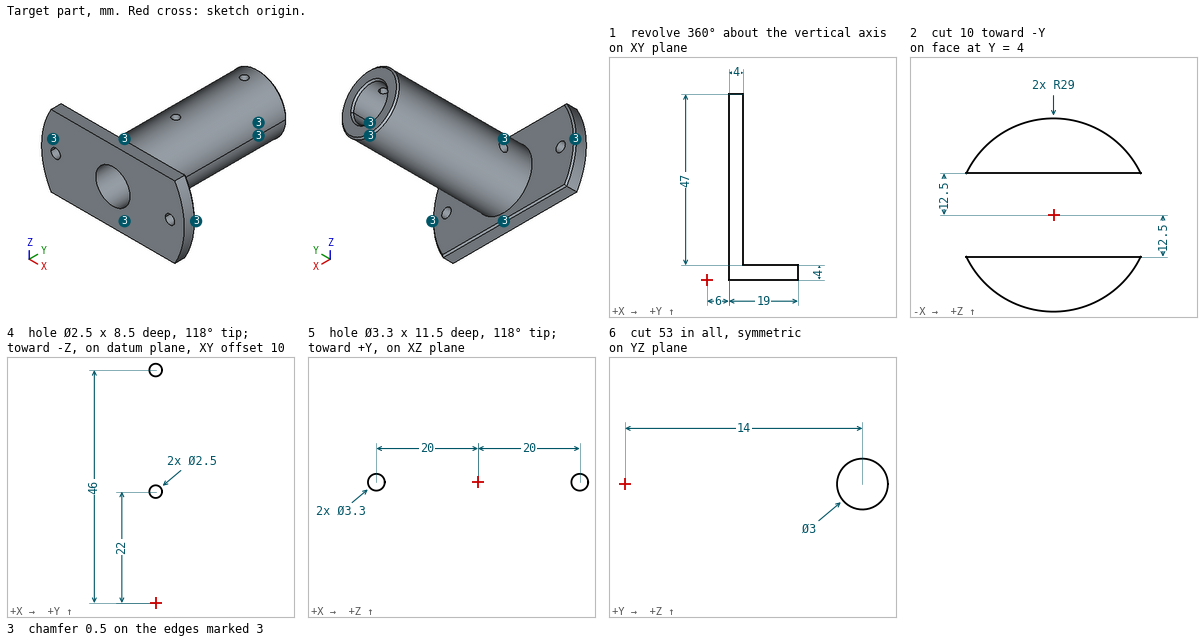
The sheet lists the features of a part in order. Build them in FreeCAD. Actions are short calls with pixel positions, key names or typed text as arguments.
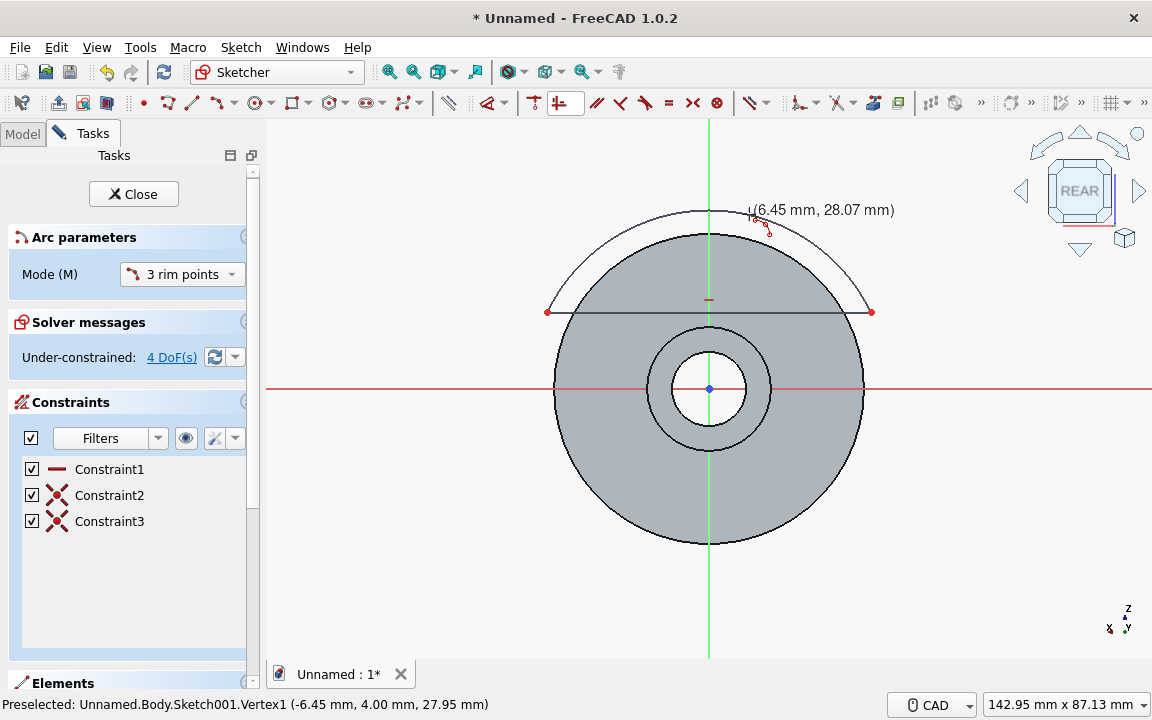
click(192, 104)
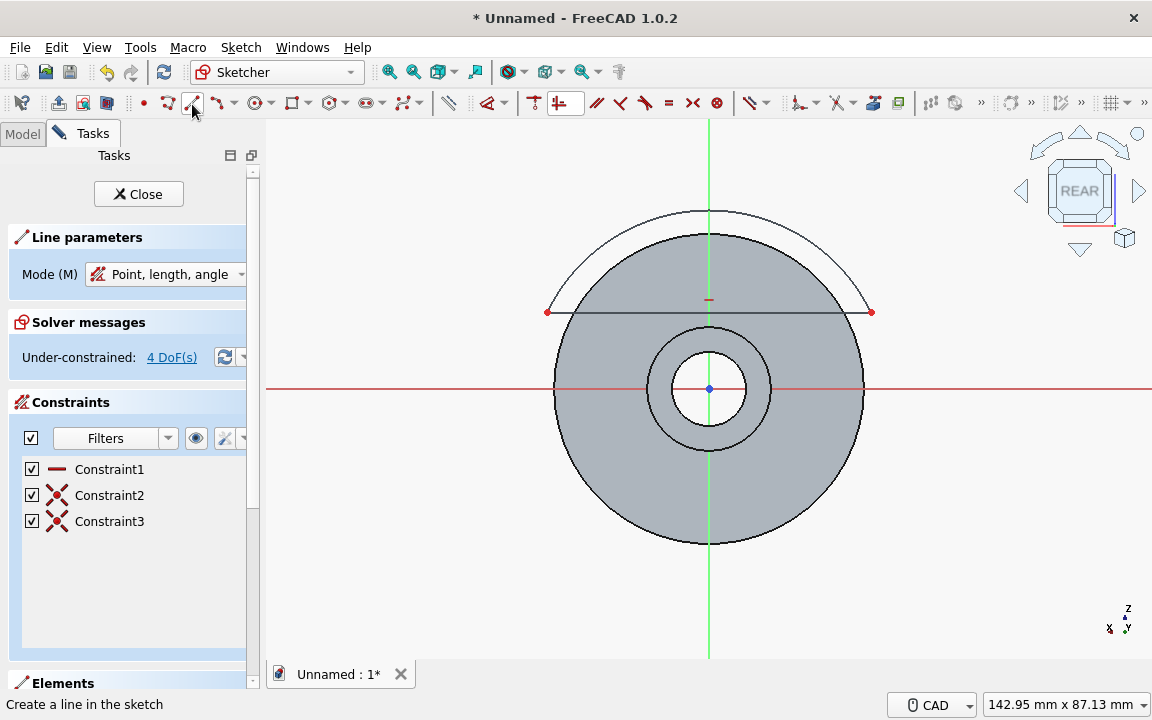
click(871, 466)
click(547, 466)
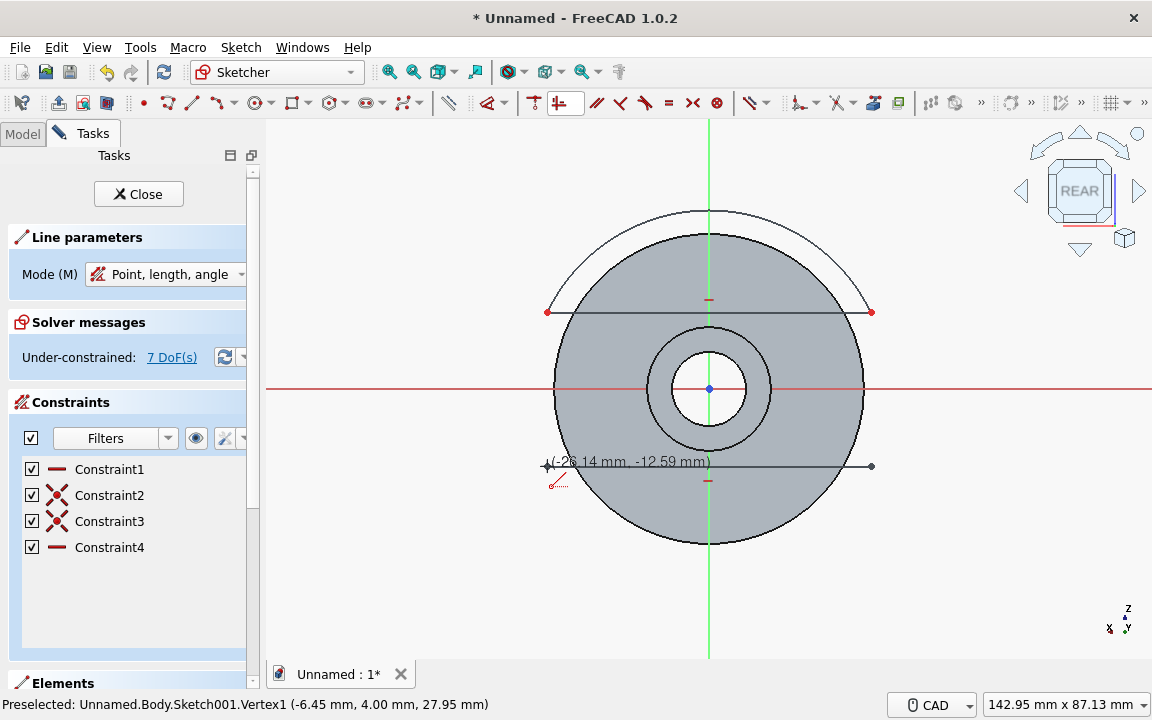
click(218, 104)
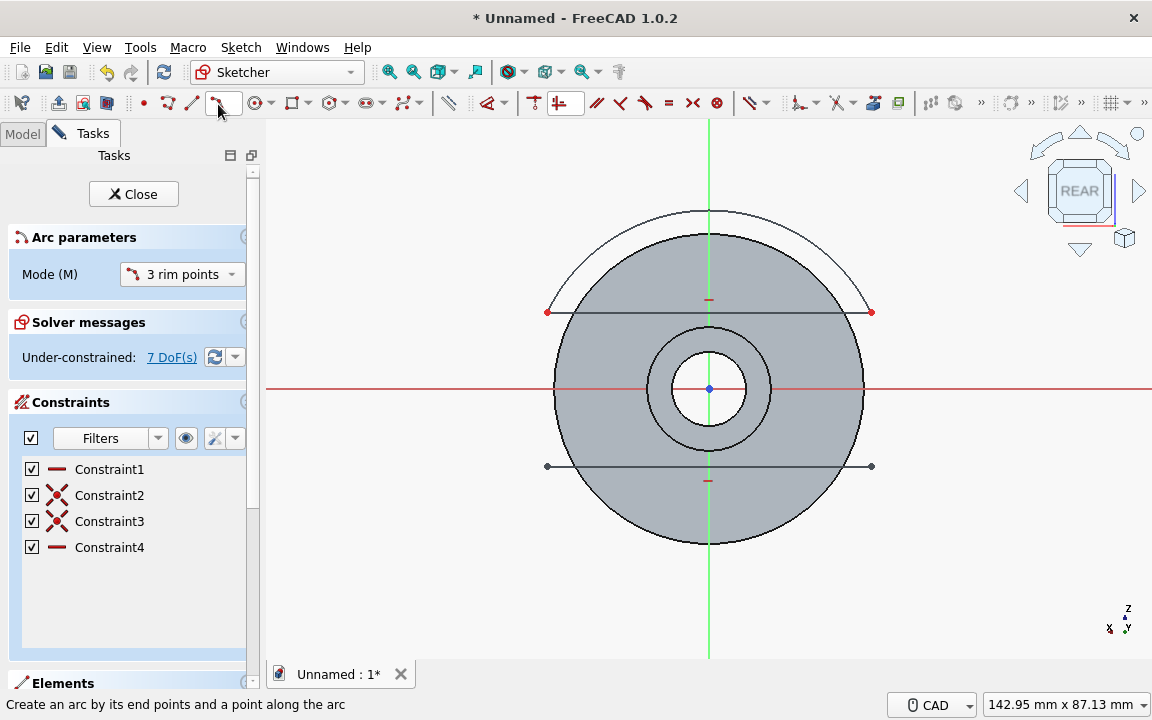
click(547, 467)
click(871, 467)
click(669, 564)
key(Escape)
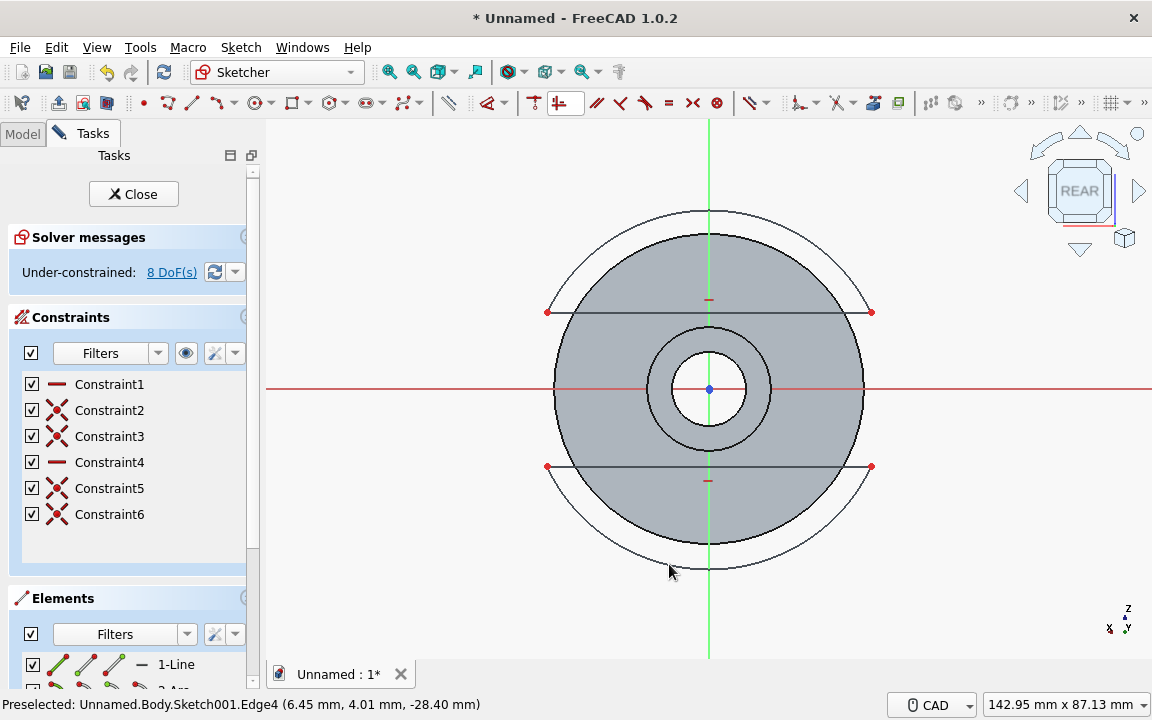
click(787, 228)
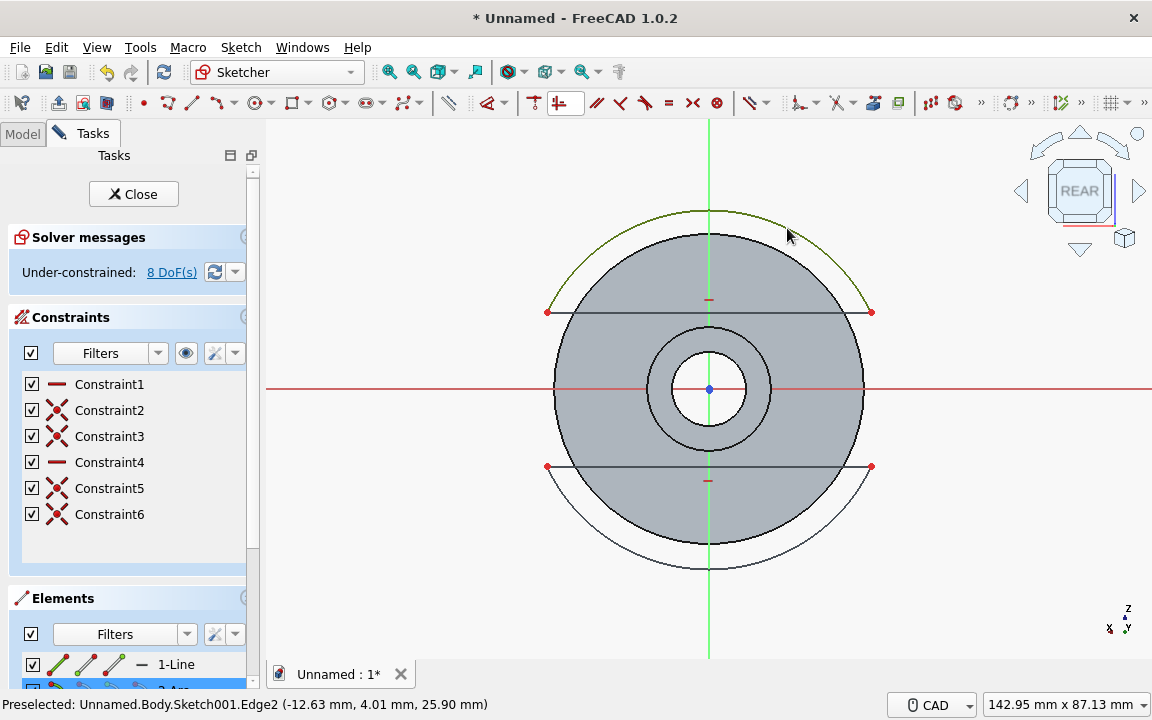
click(631, 552)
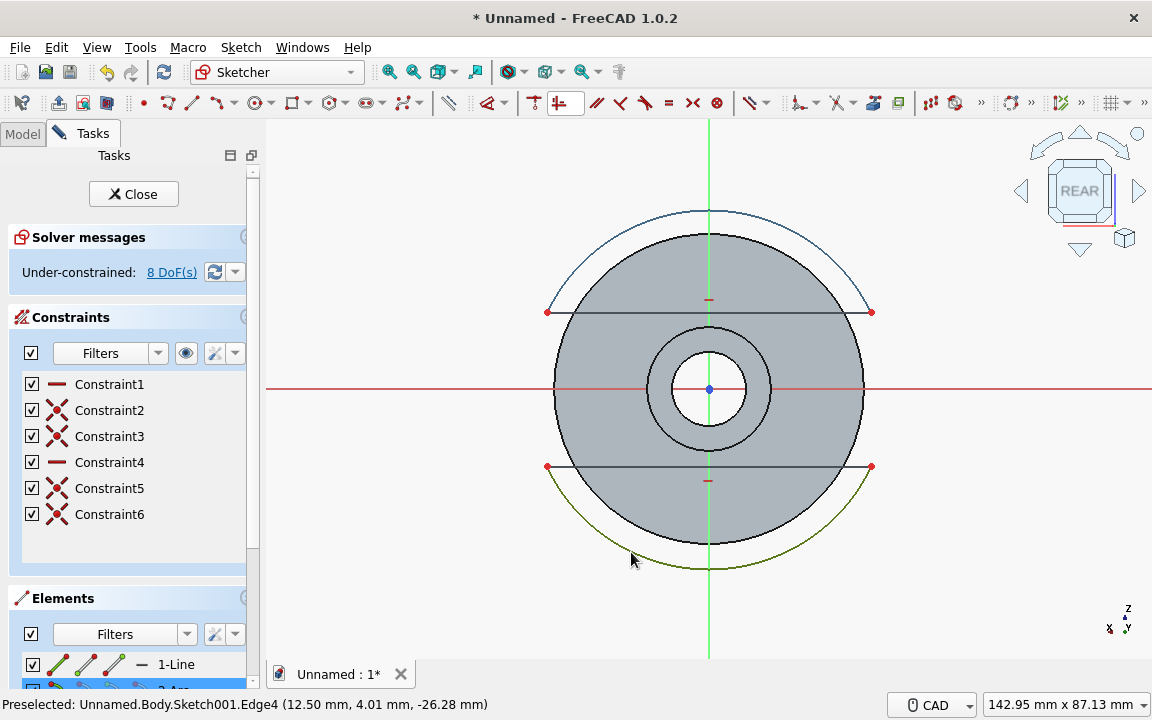
click(534, 104)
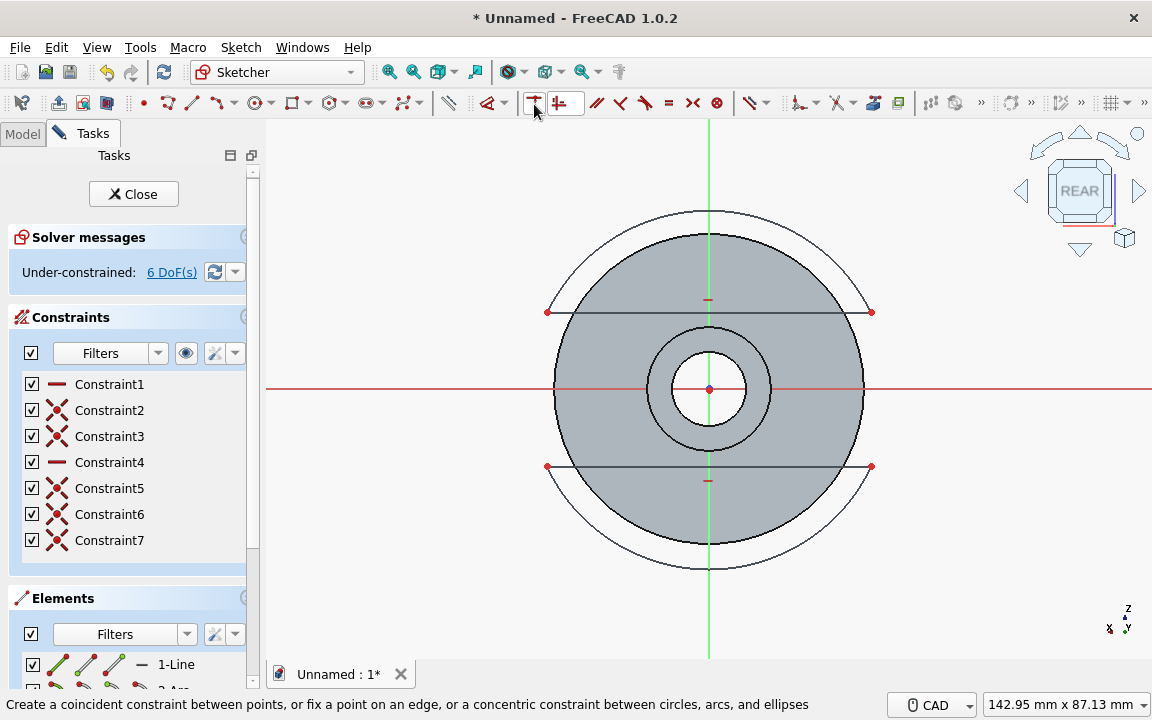
drag(699, 379, 719, 400)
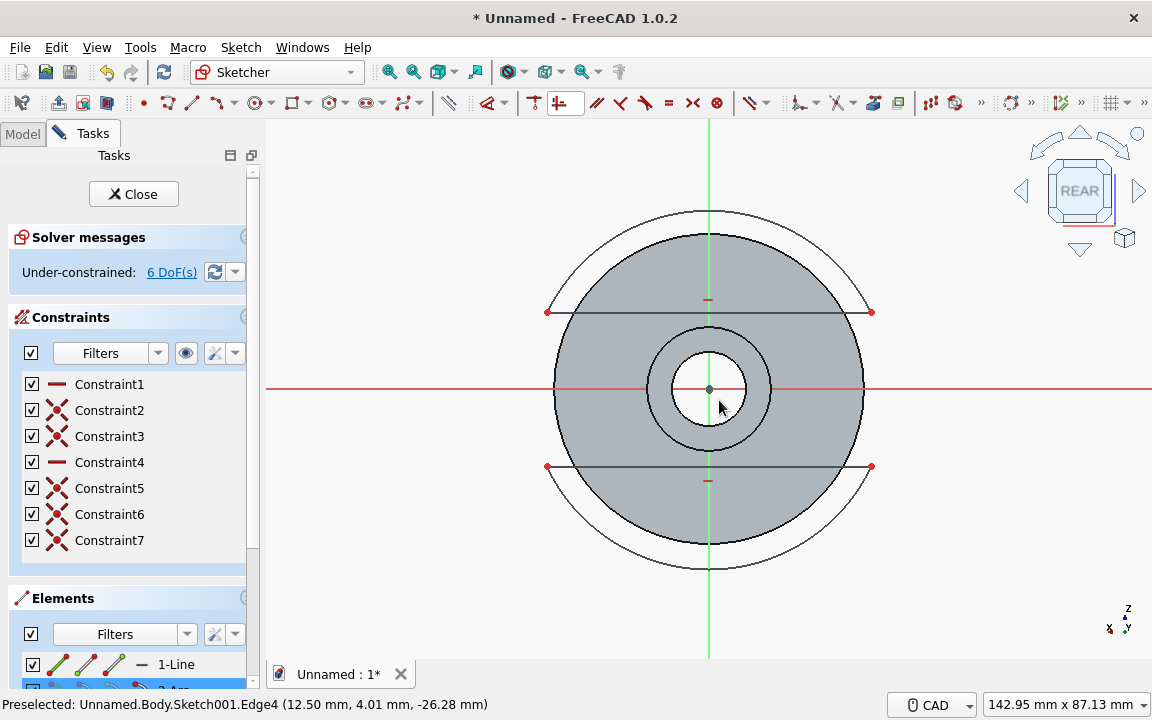
click(534, 104)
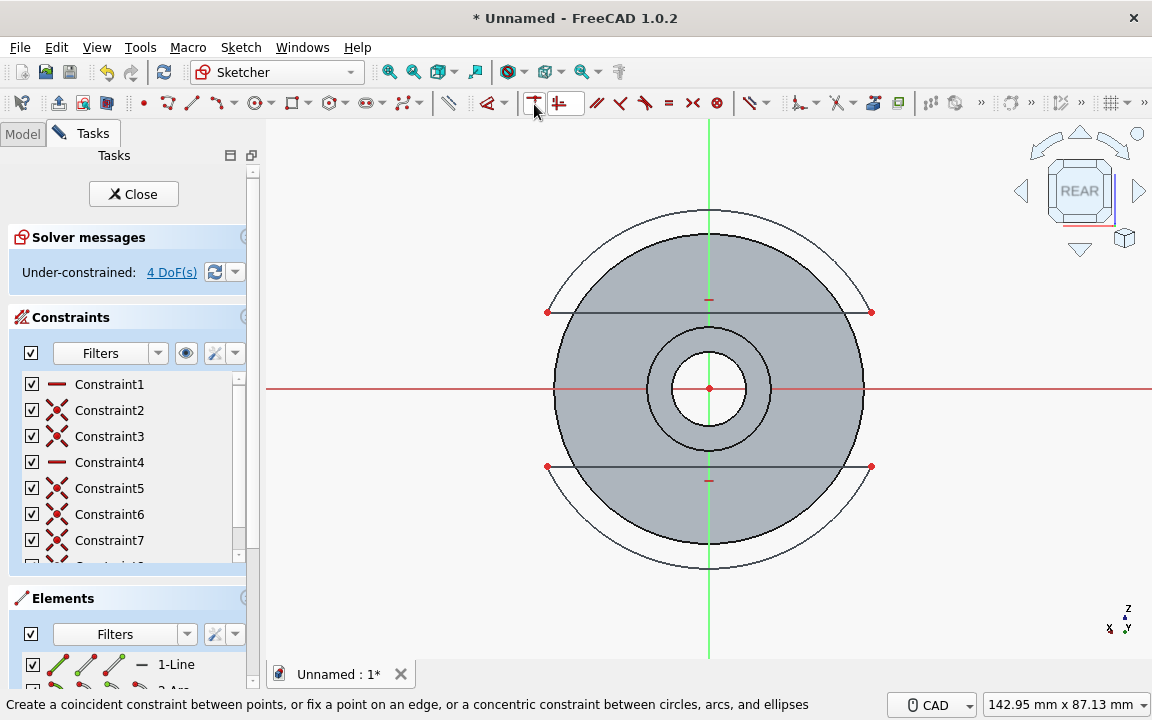
click(787, 228)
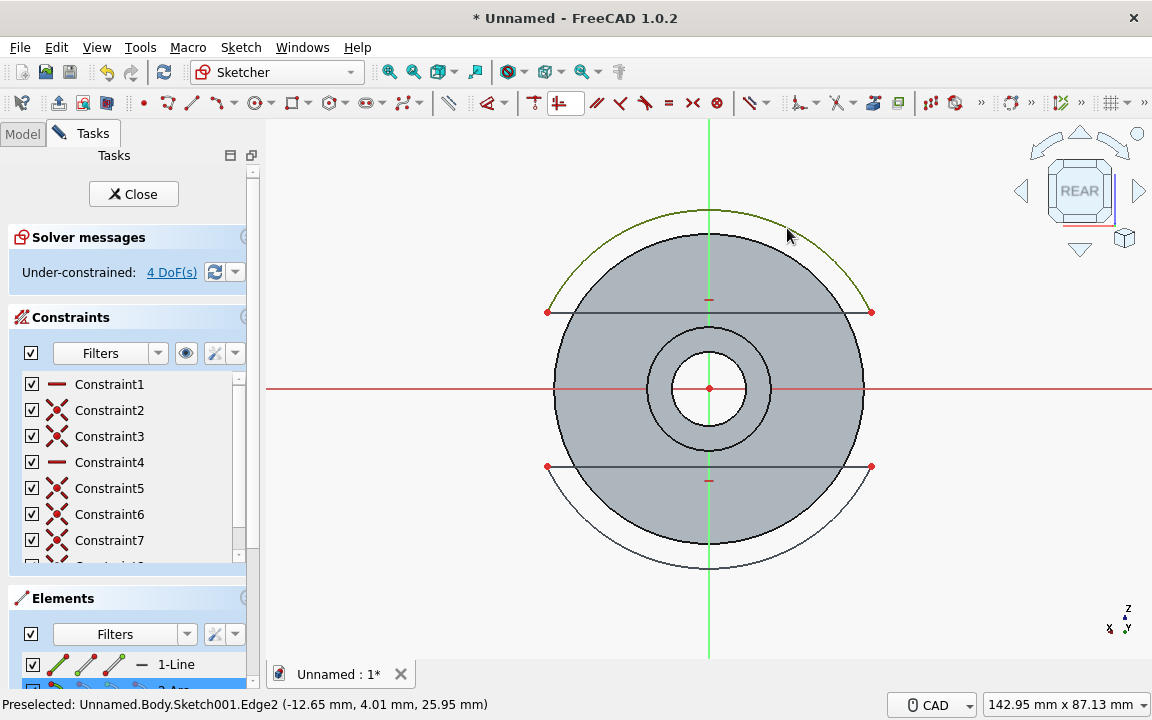
click(631, 551)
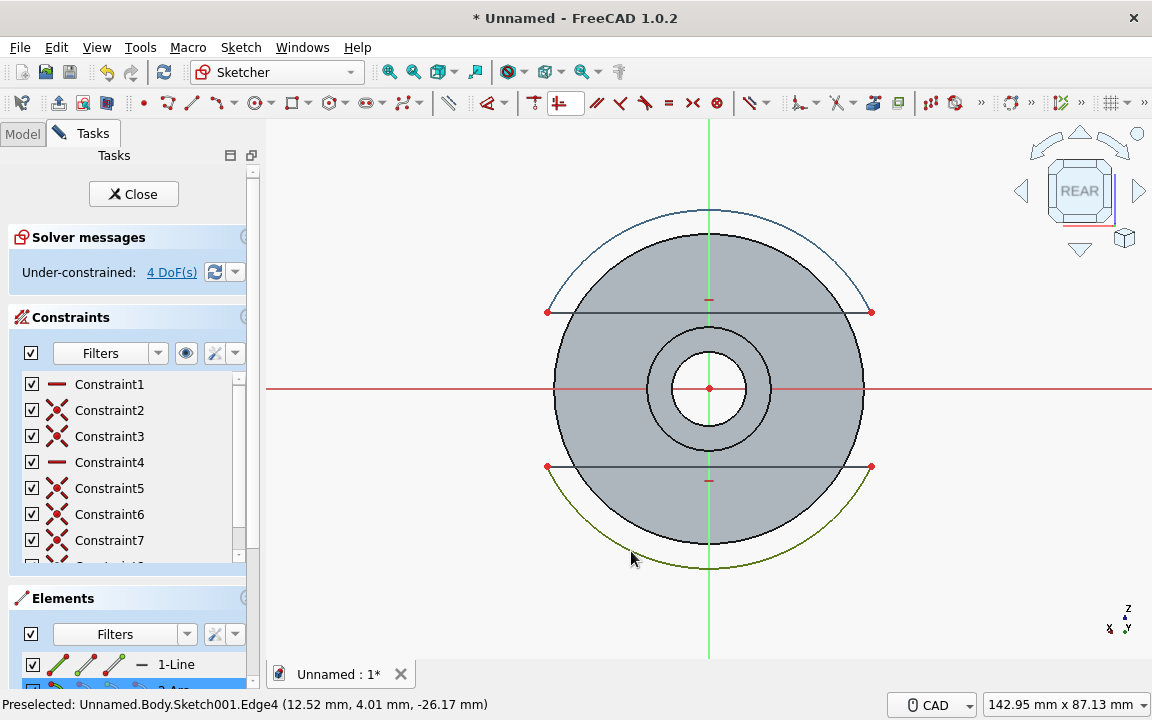
click(670, 104)